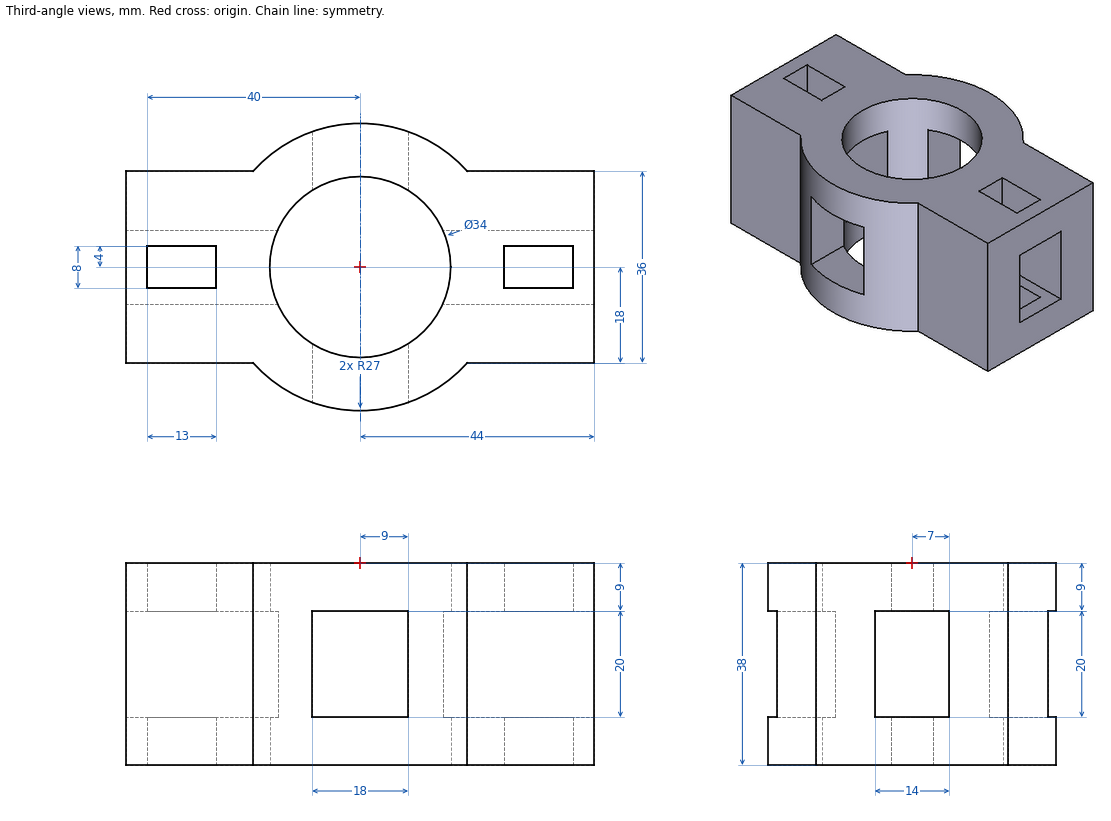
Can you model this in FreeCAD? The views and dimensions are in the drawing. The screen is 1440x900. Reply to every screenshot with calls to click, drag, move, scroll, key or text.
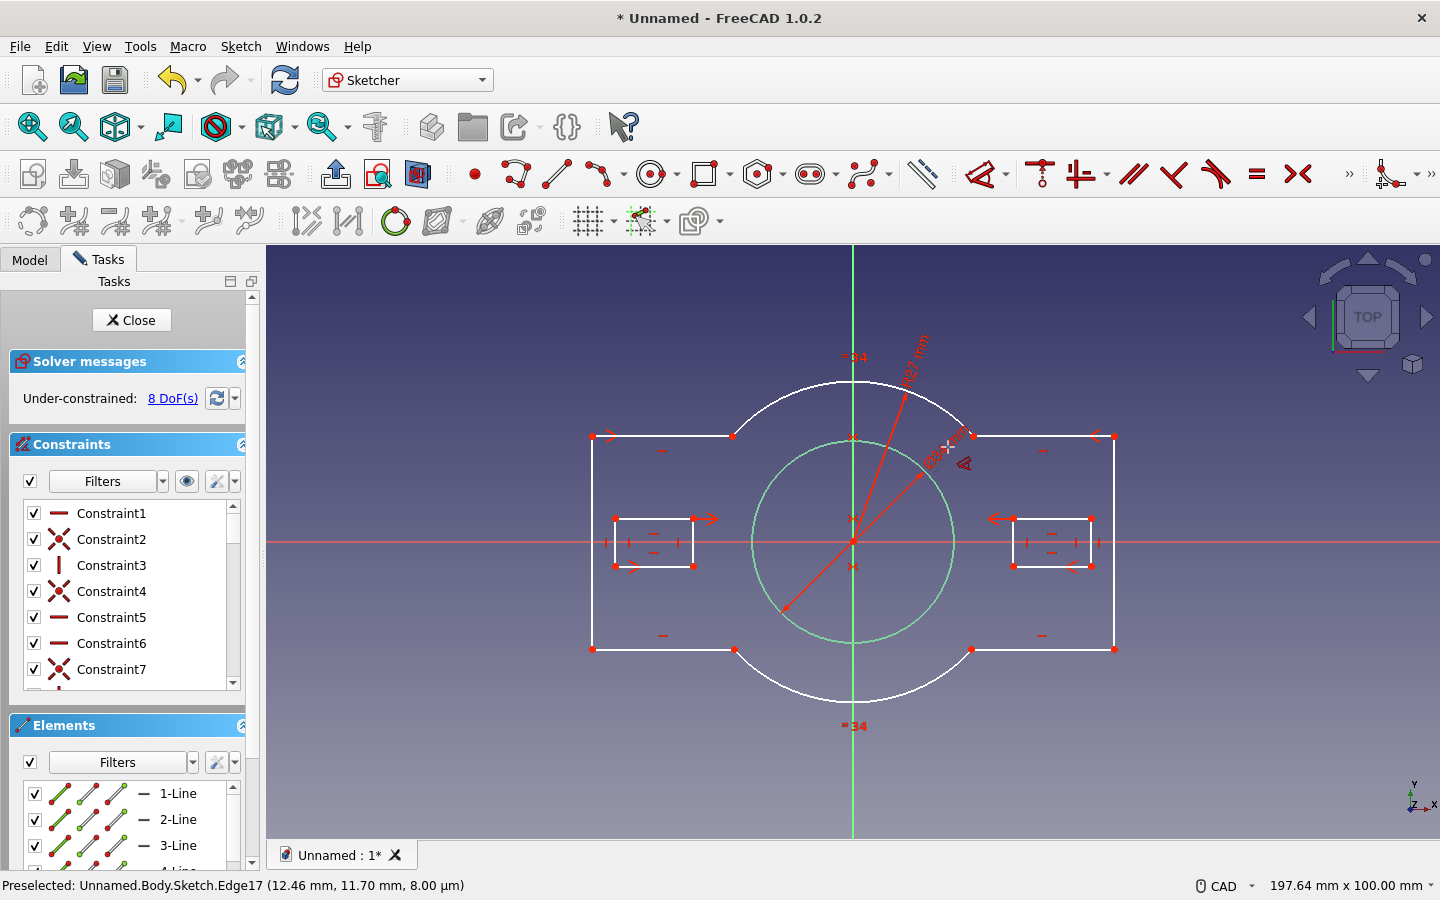
scroll(615, 553, up, 2)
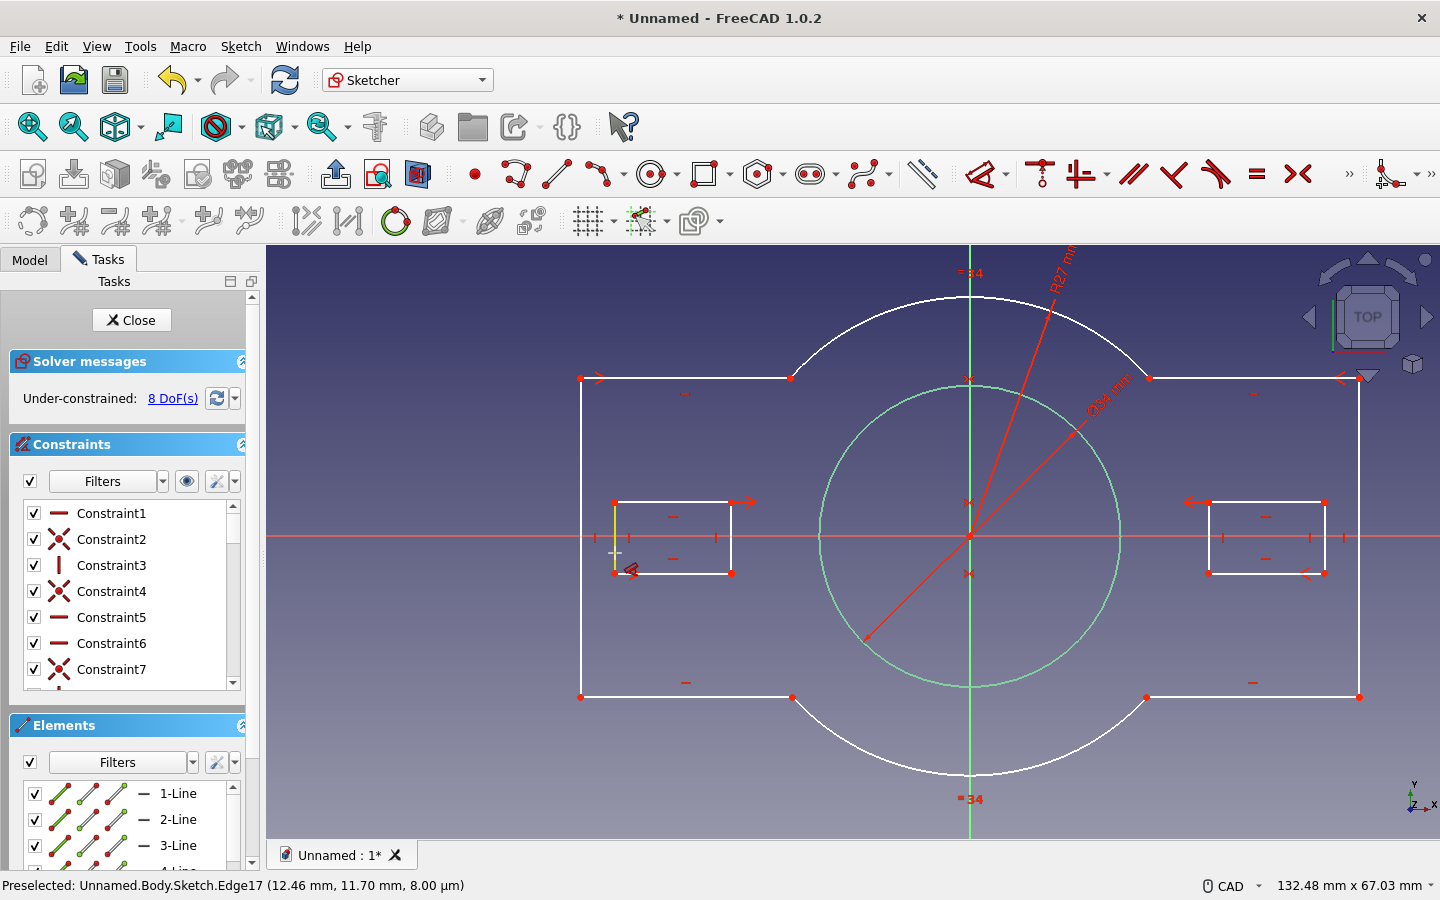
click(615, 552)
click(649, 521)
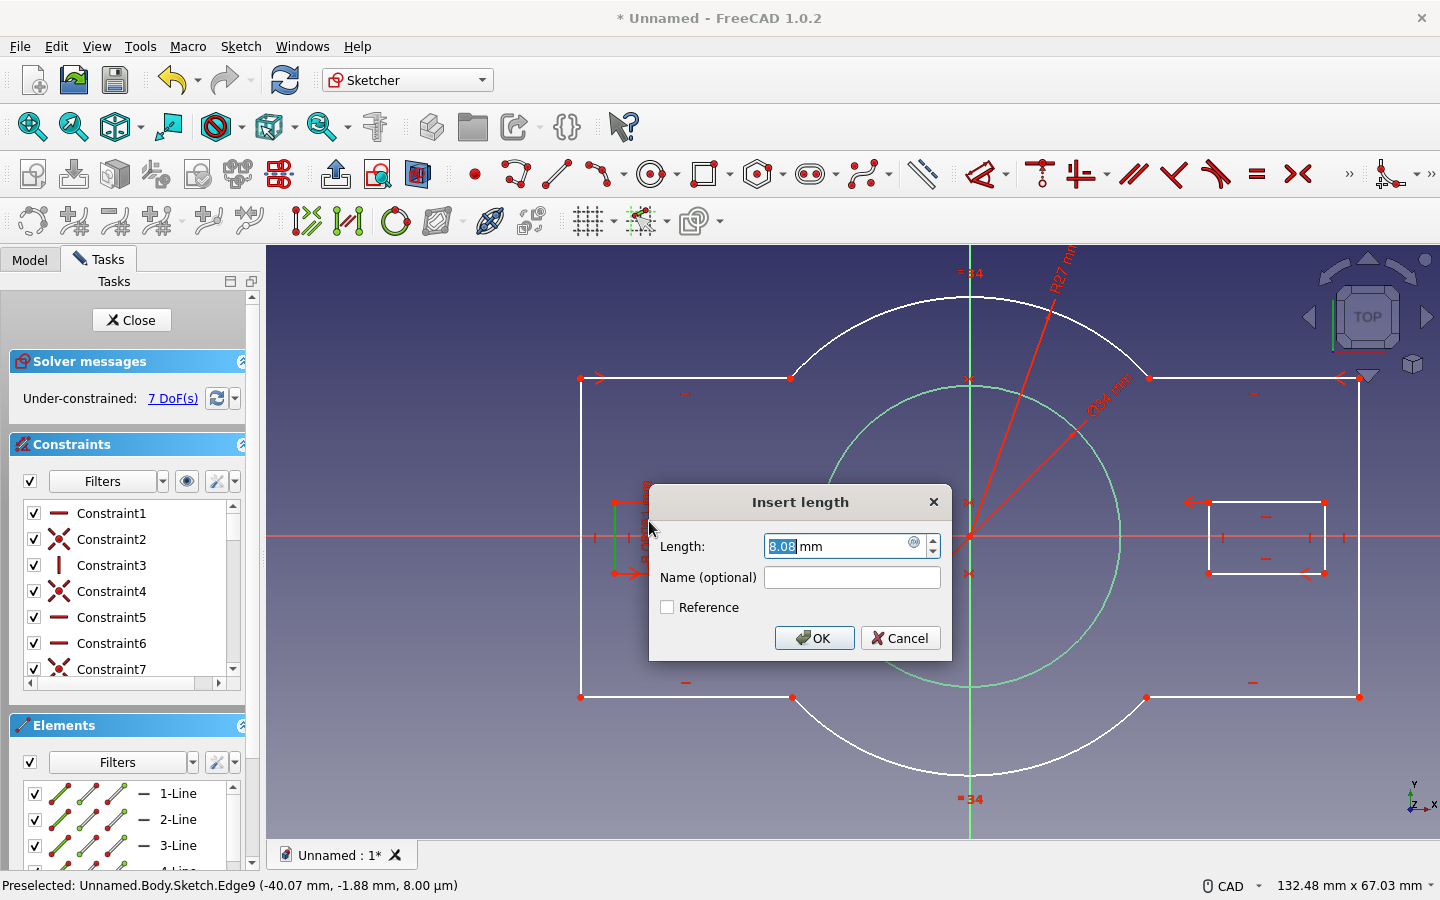
text(8)
key(Return)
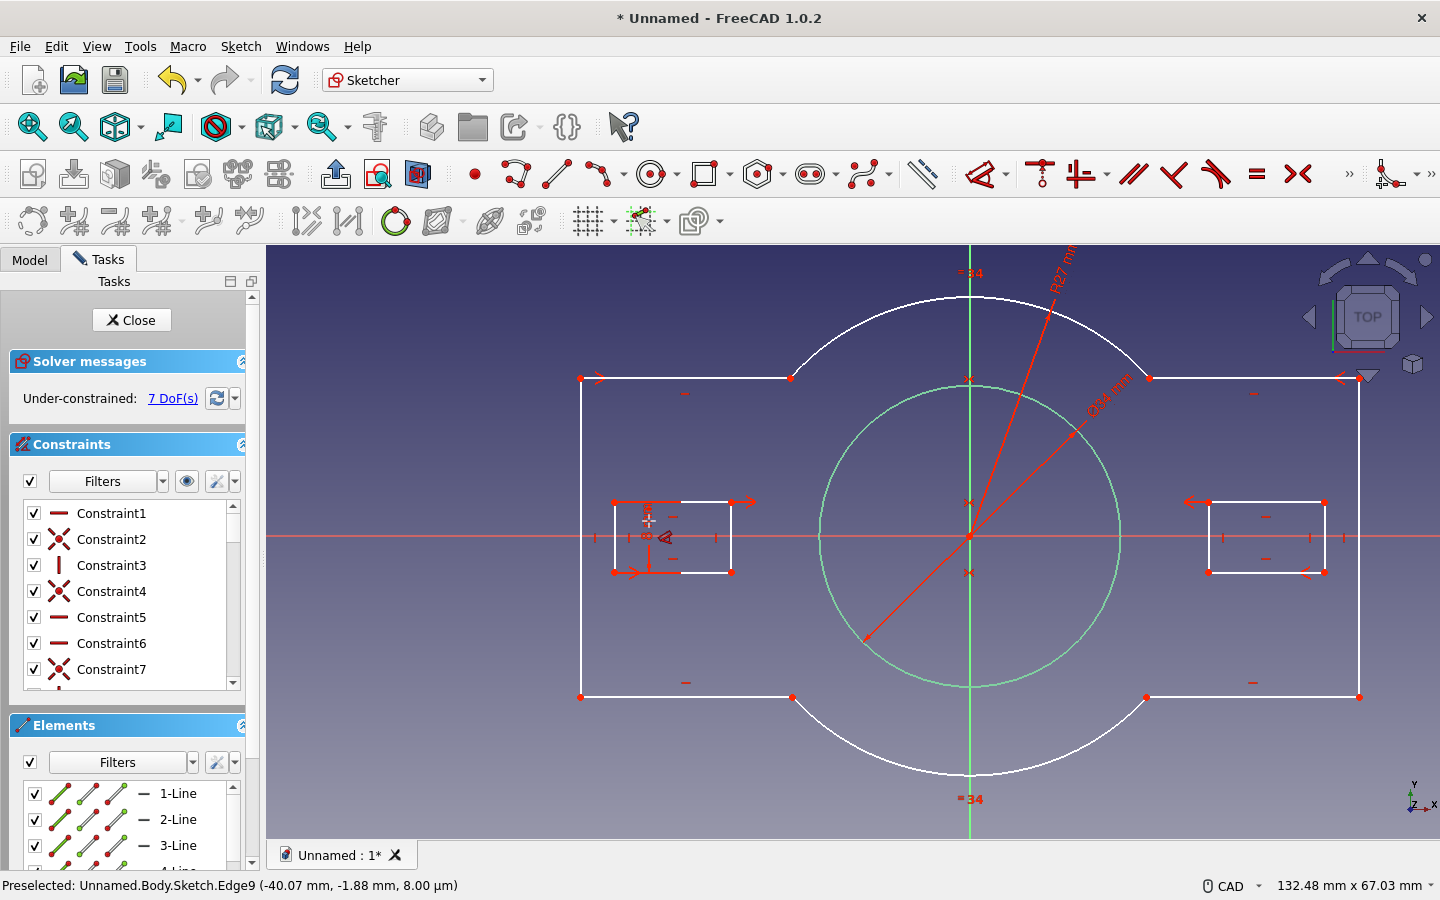
scroll(294, 568, down, 1)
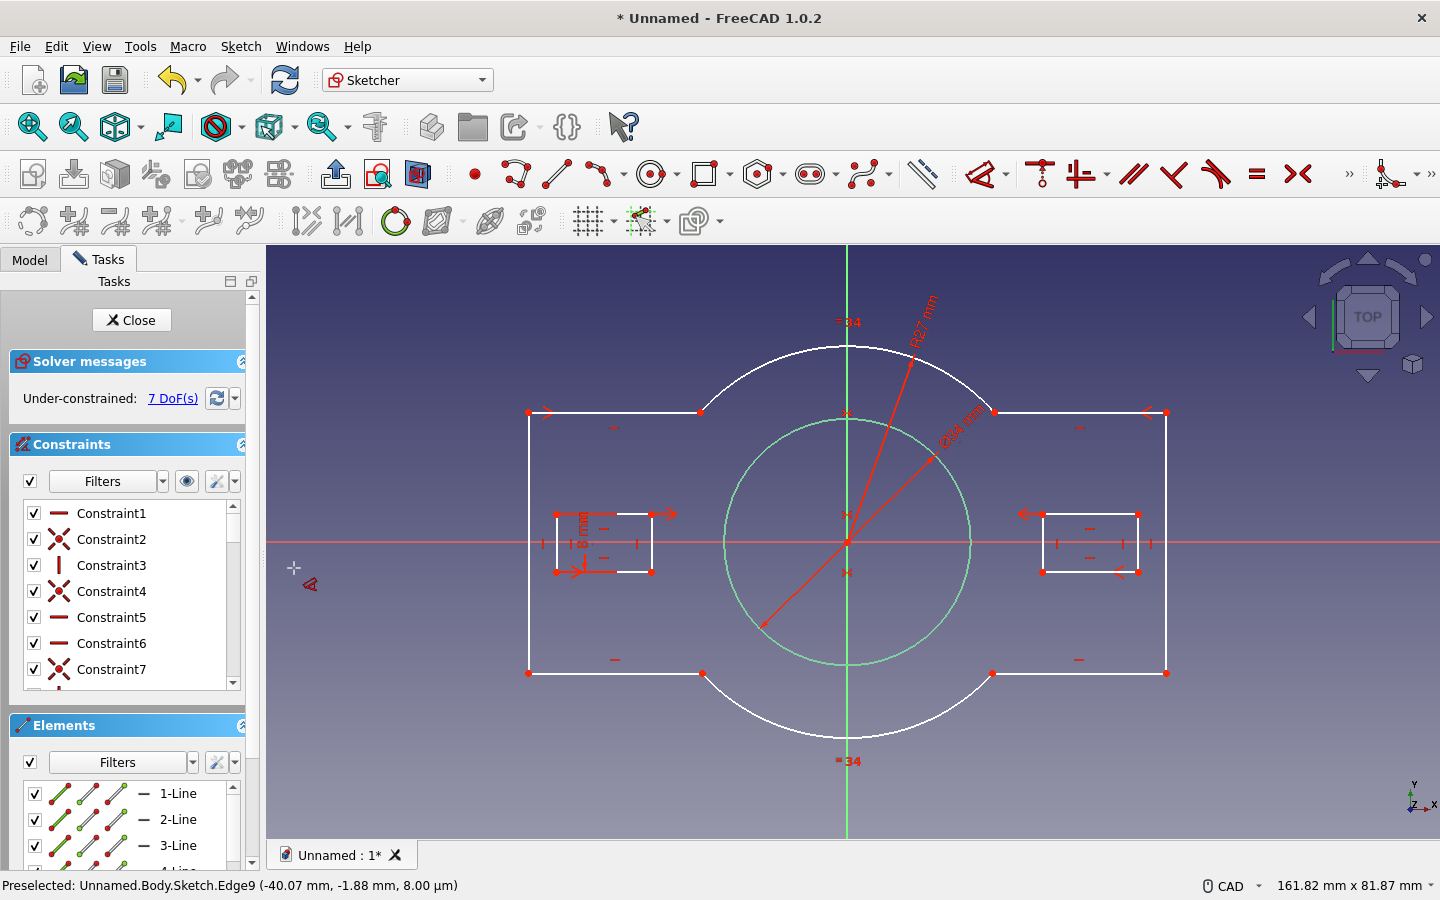
click(1166, 596)
click(1200, 483)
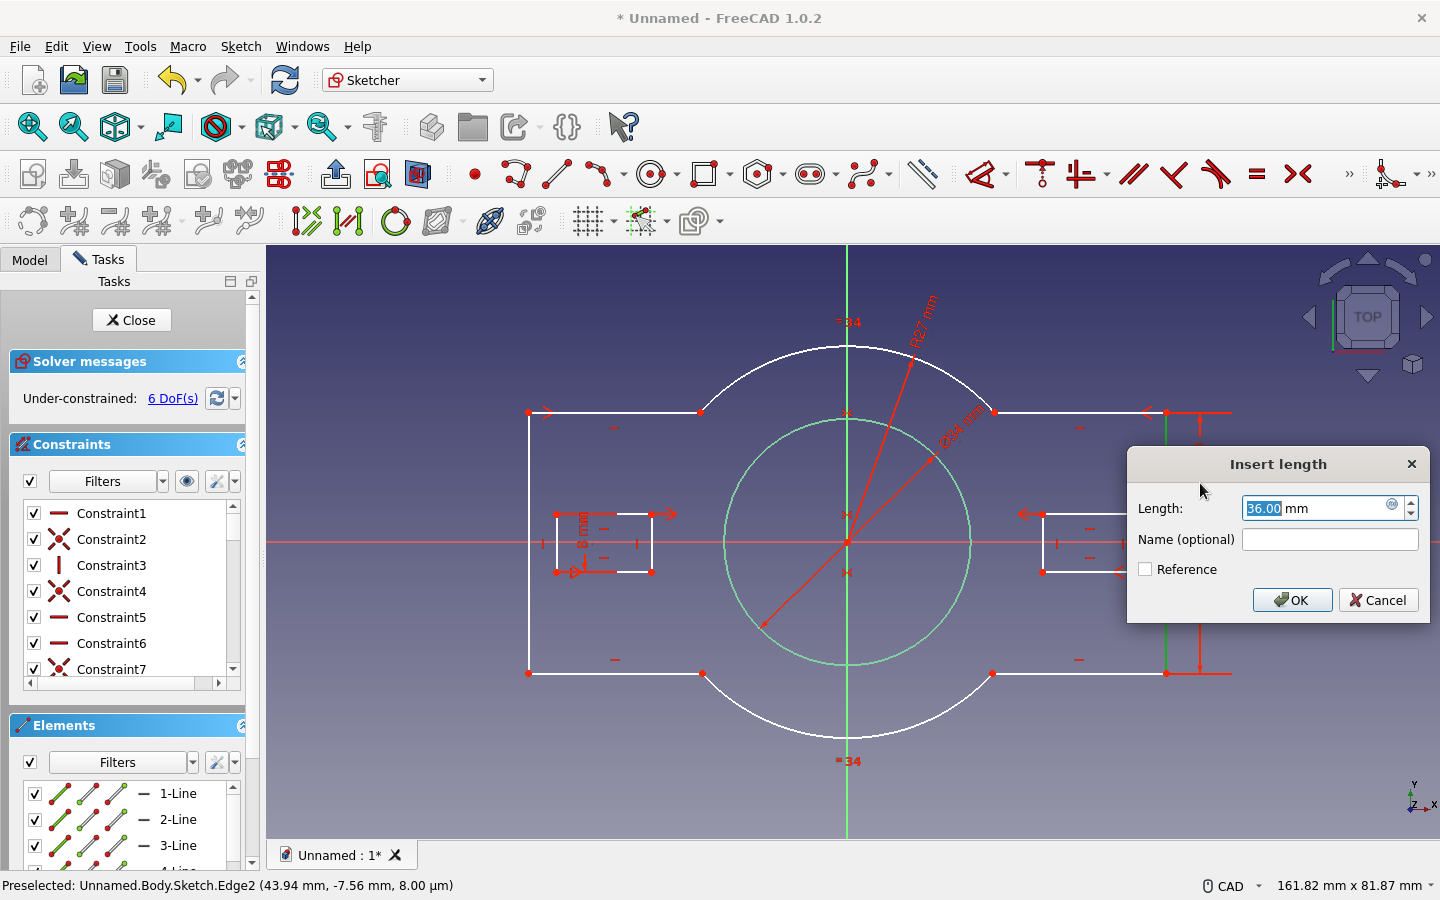
text(36)
key(Return)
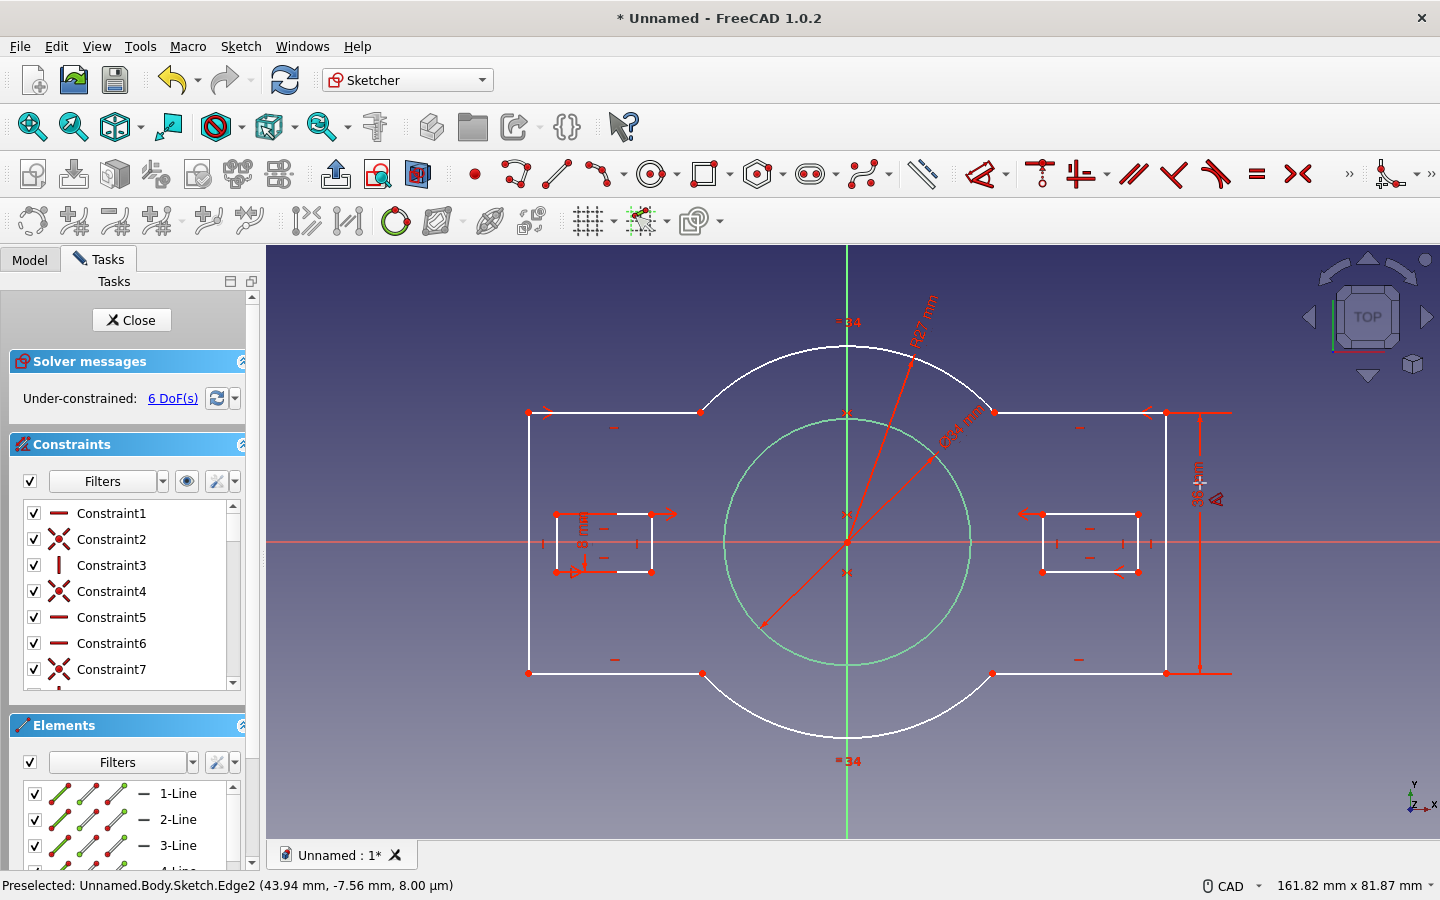
click(529, 491)
click(495, 483)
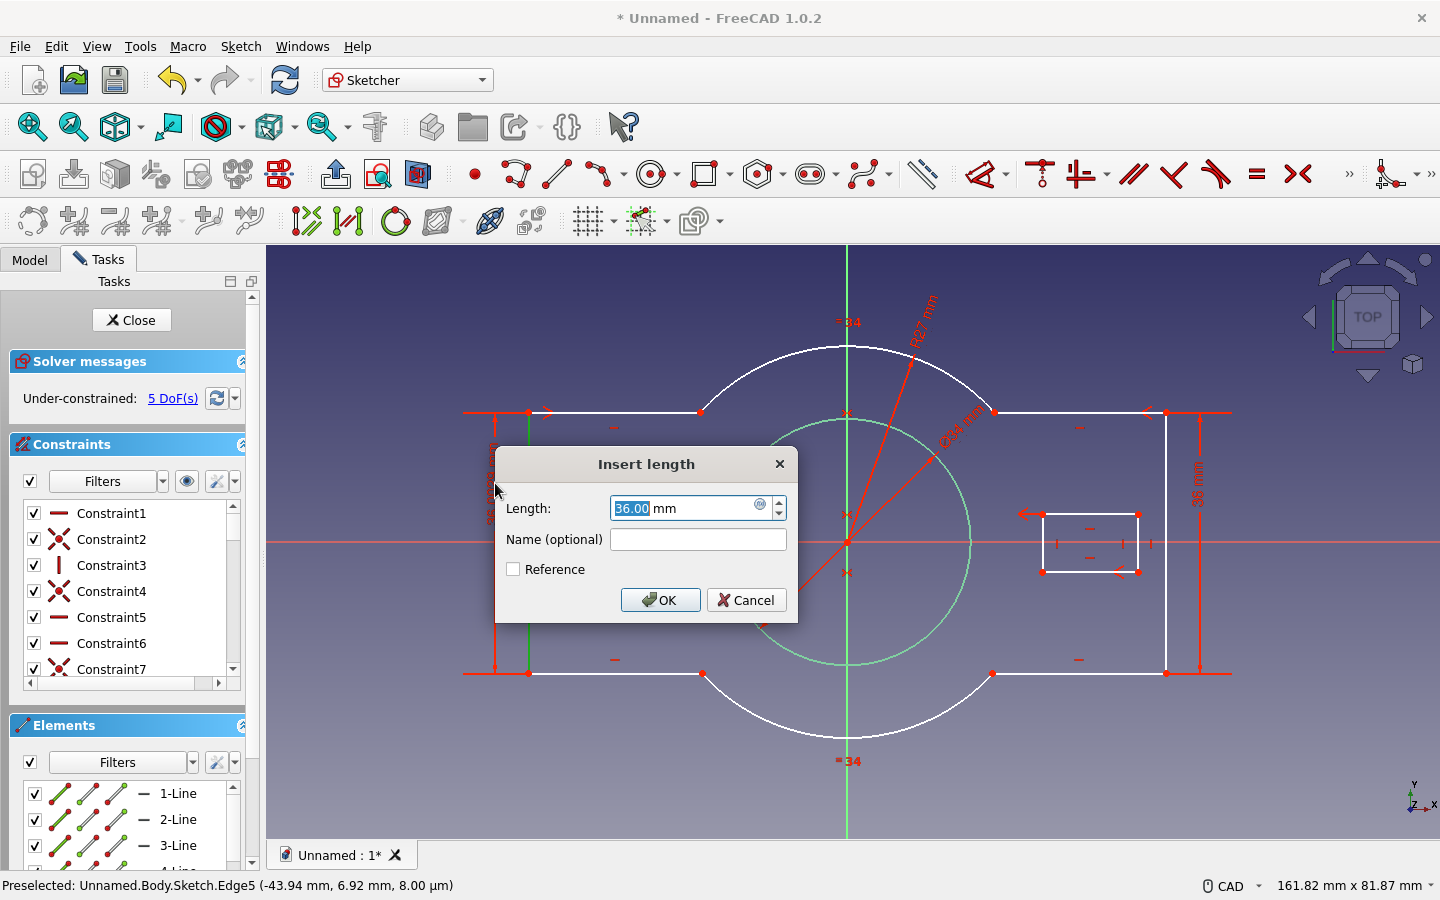
text(36)
key(Return)